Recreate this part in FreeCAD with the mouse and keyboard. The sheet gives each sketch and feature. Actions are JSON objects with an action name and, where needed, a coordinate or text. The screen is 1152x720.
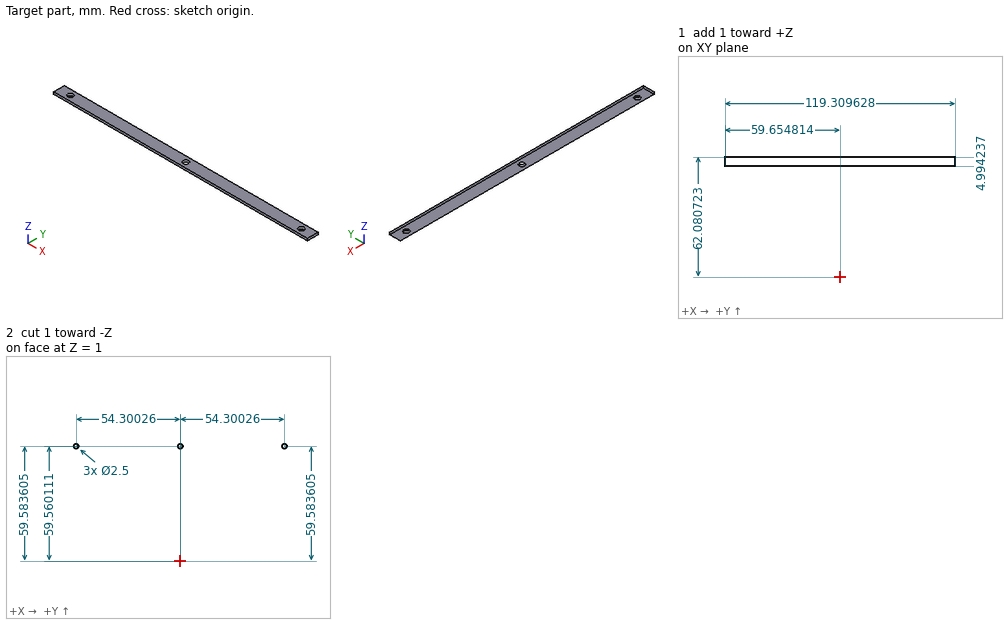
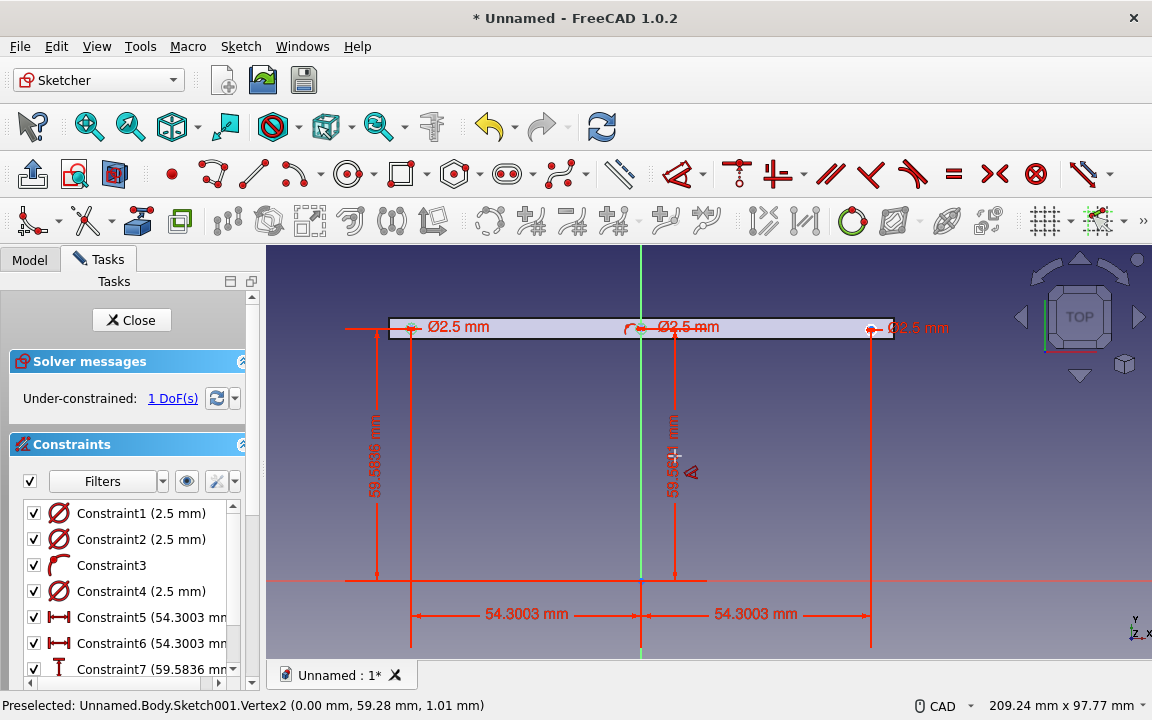
{"action": "left_click", "coordinate": [871, 330]}
{"action": "left_click", "coordinate": [905, 456]}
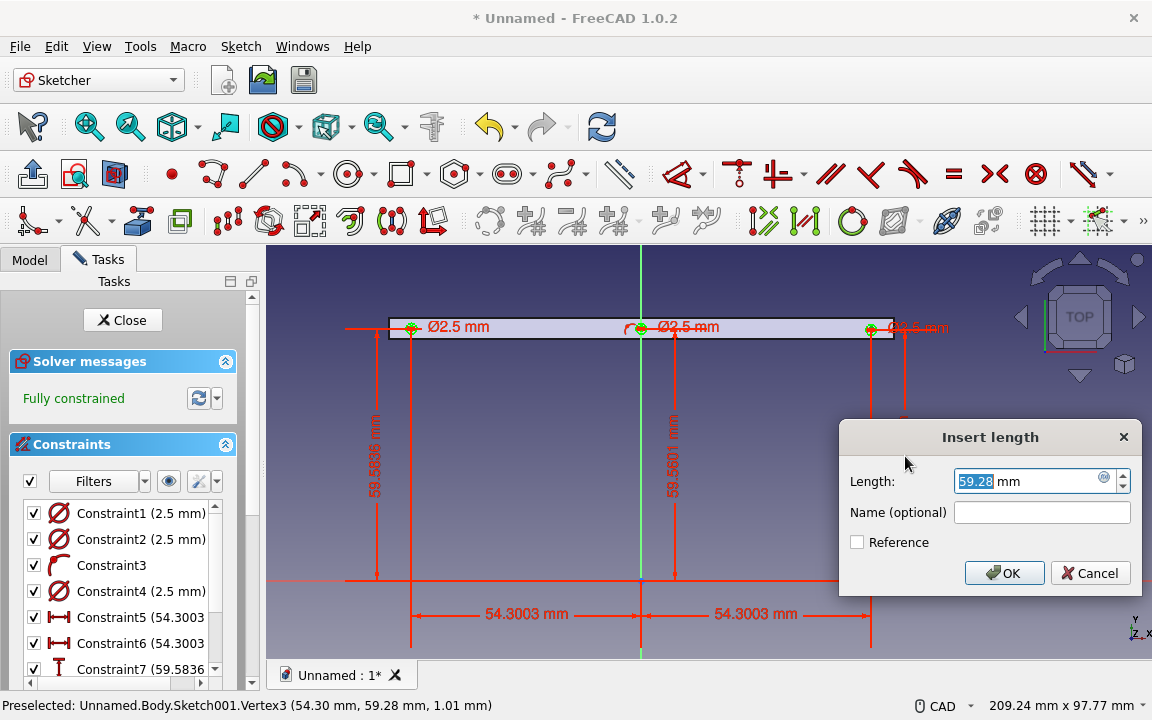
{"action": "type", "text": "59.583605"}
{"action": "key", "text": "Return"}
{"action": "key", "text": "Escape"}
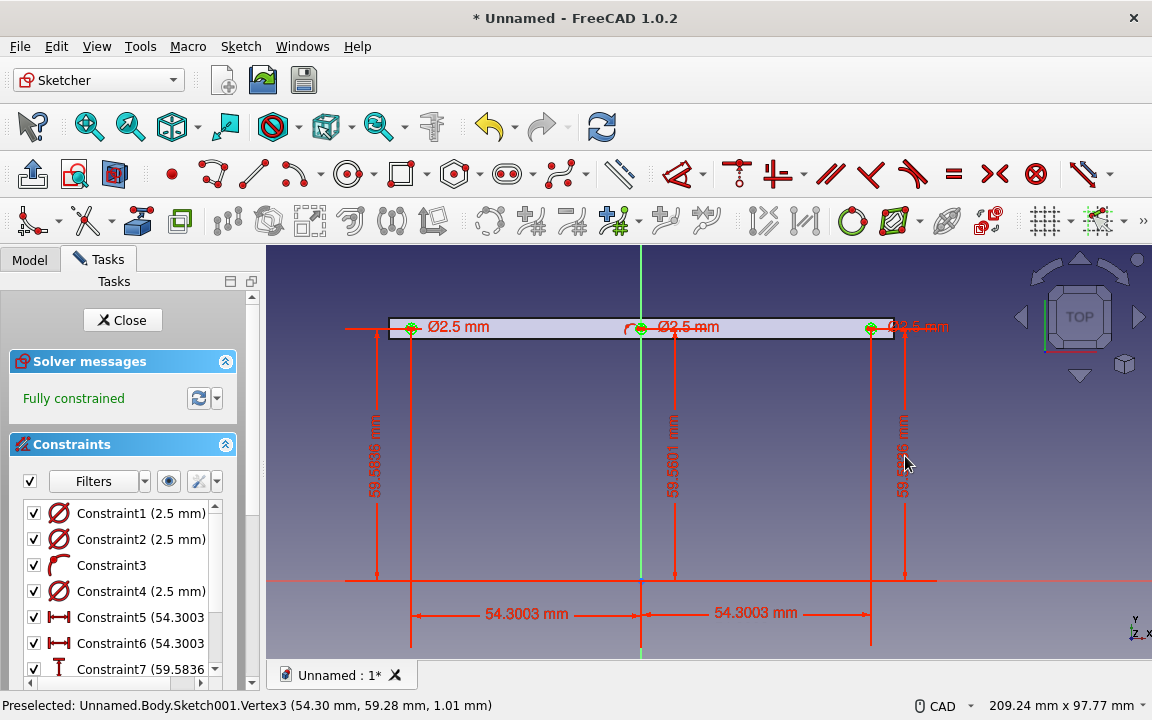
{"action": "left_click", "coordinate": [123, 320]}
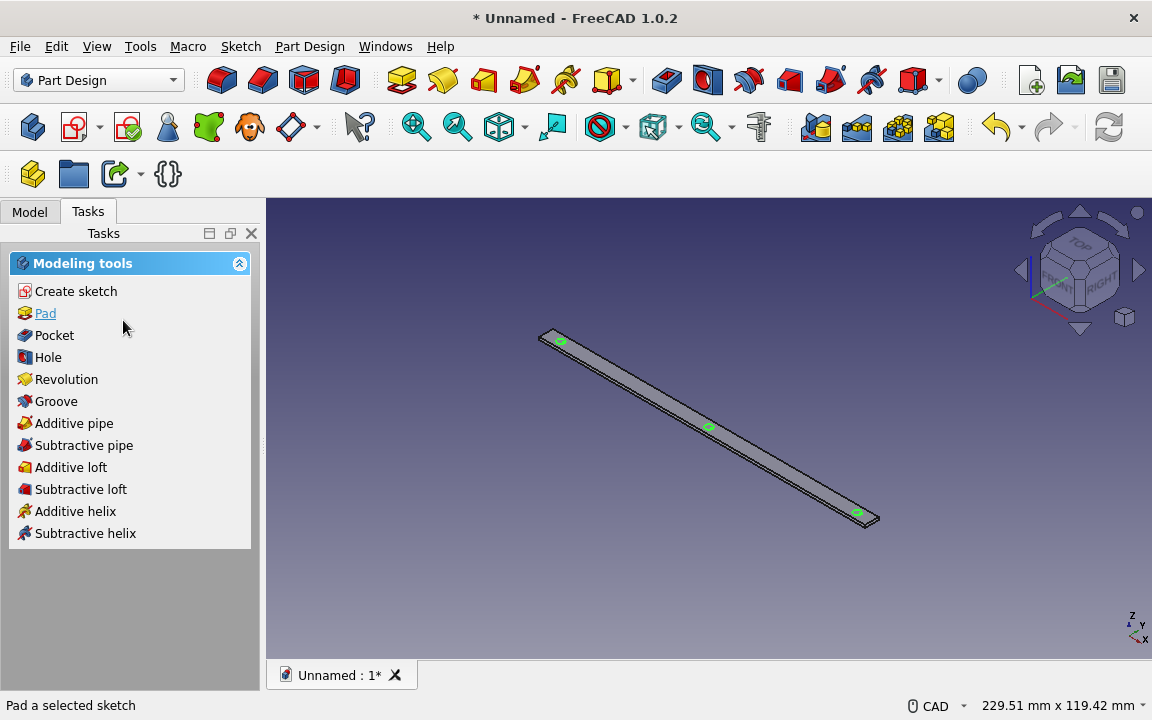
{"action": "left_click", "coordinate": [667, 80]}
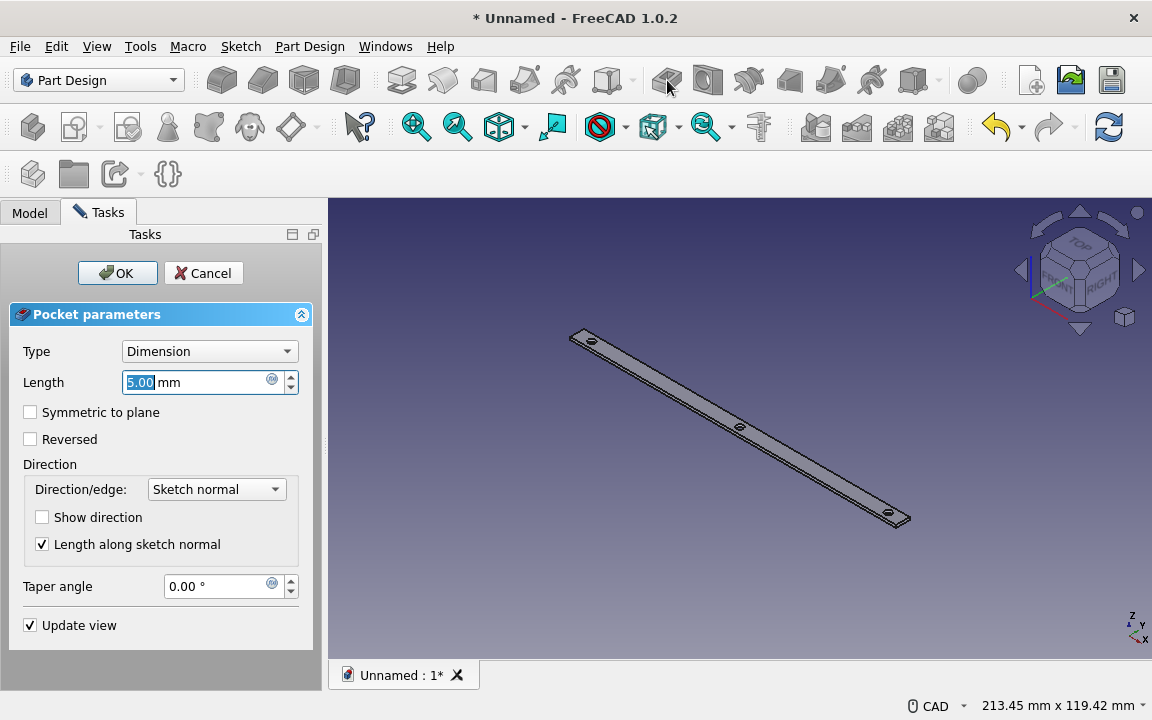
{"action": "type", "text": "1"}
{"action": "key", "text": "Tab"}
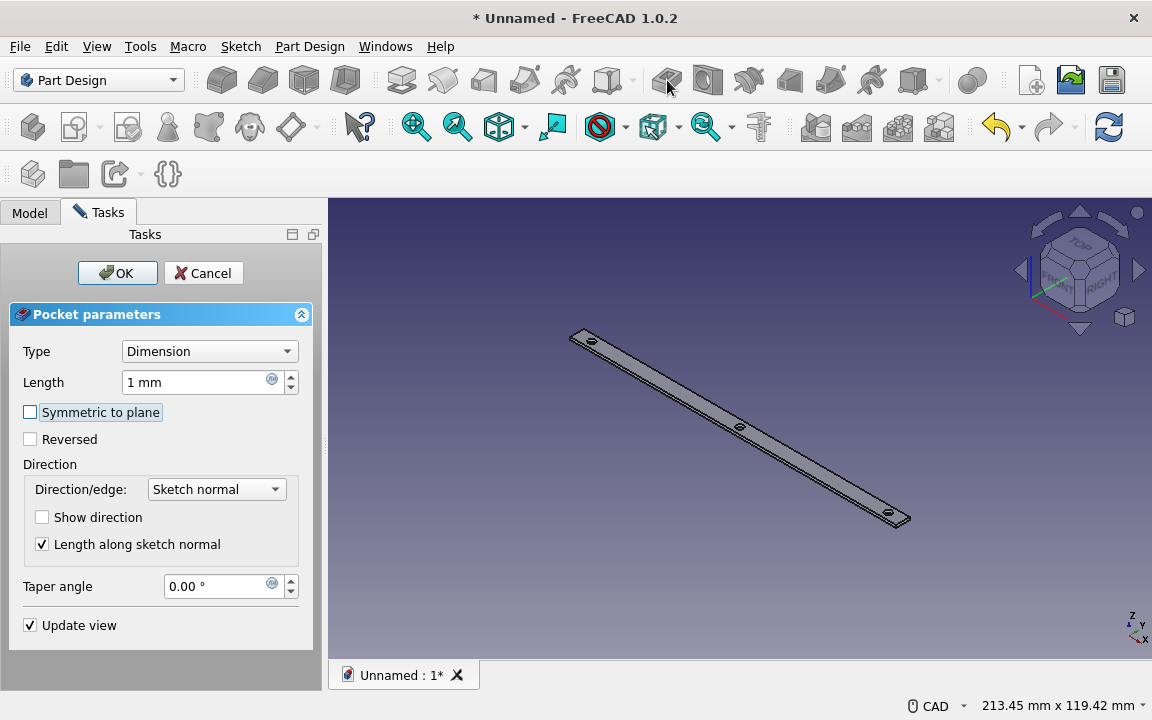
{"action": "left_click", "coordinate": [118, 273]}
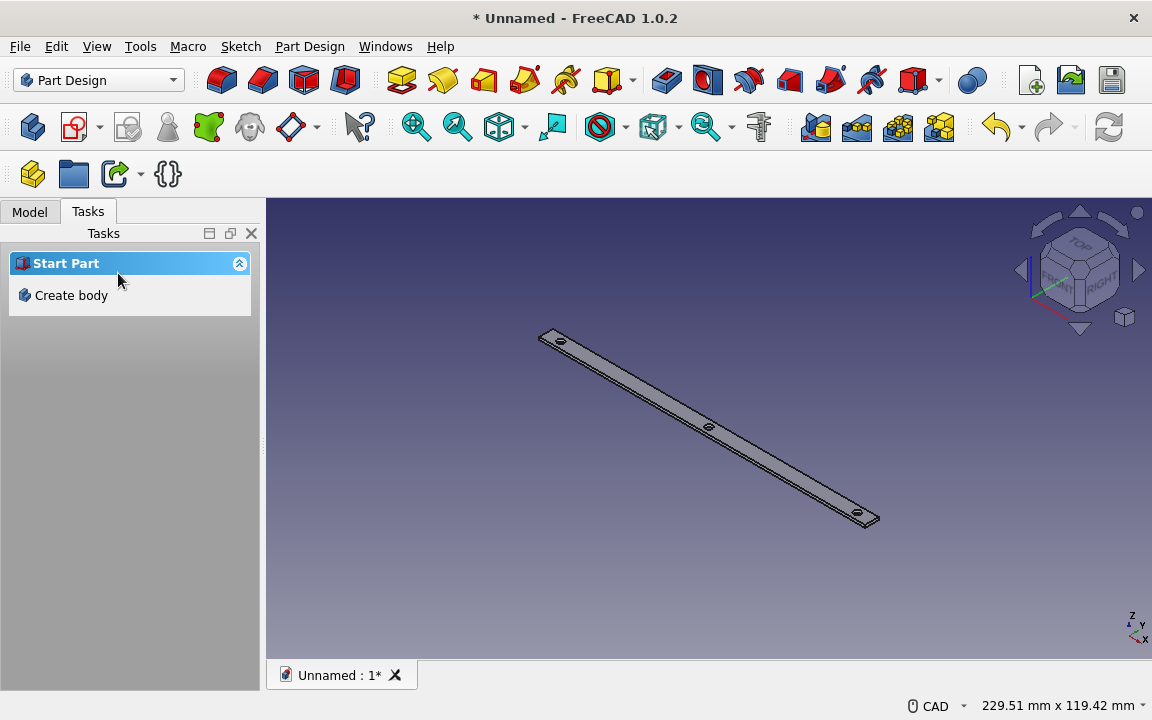
{"action": "key", "text": "v f"}